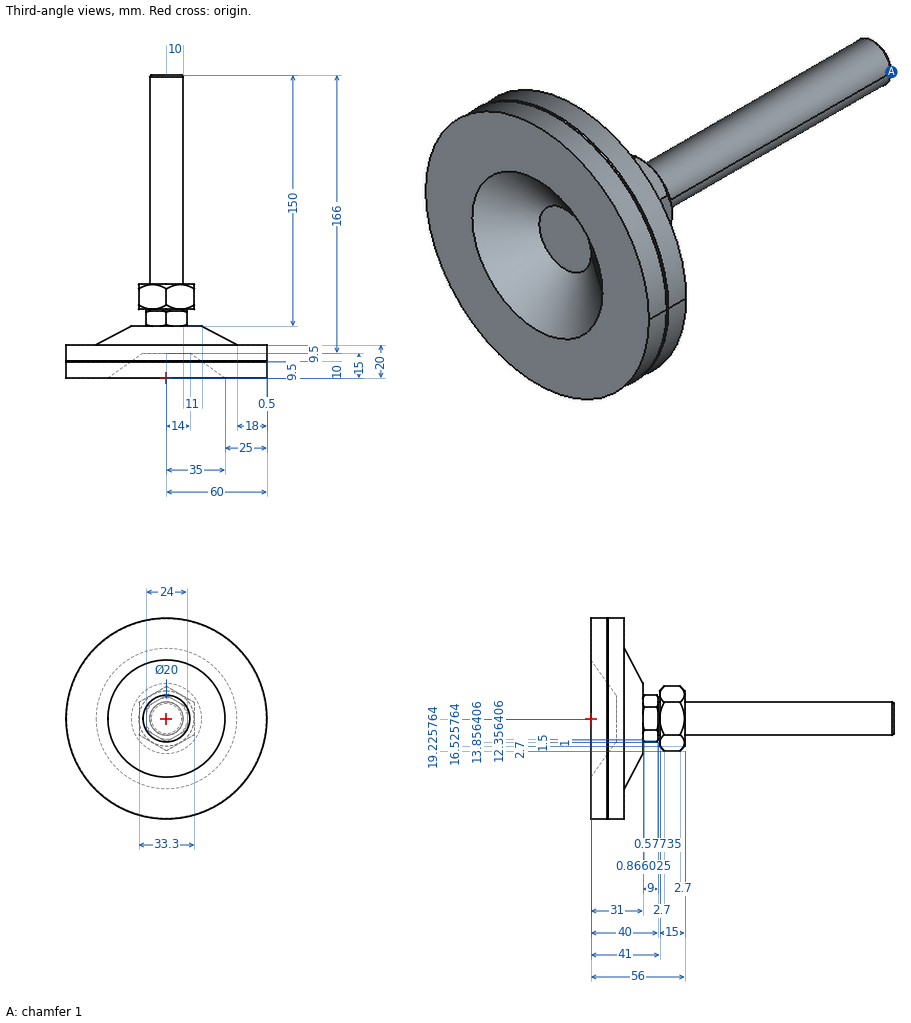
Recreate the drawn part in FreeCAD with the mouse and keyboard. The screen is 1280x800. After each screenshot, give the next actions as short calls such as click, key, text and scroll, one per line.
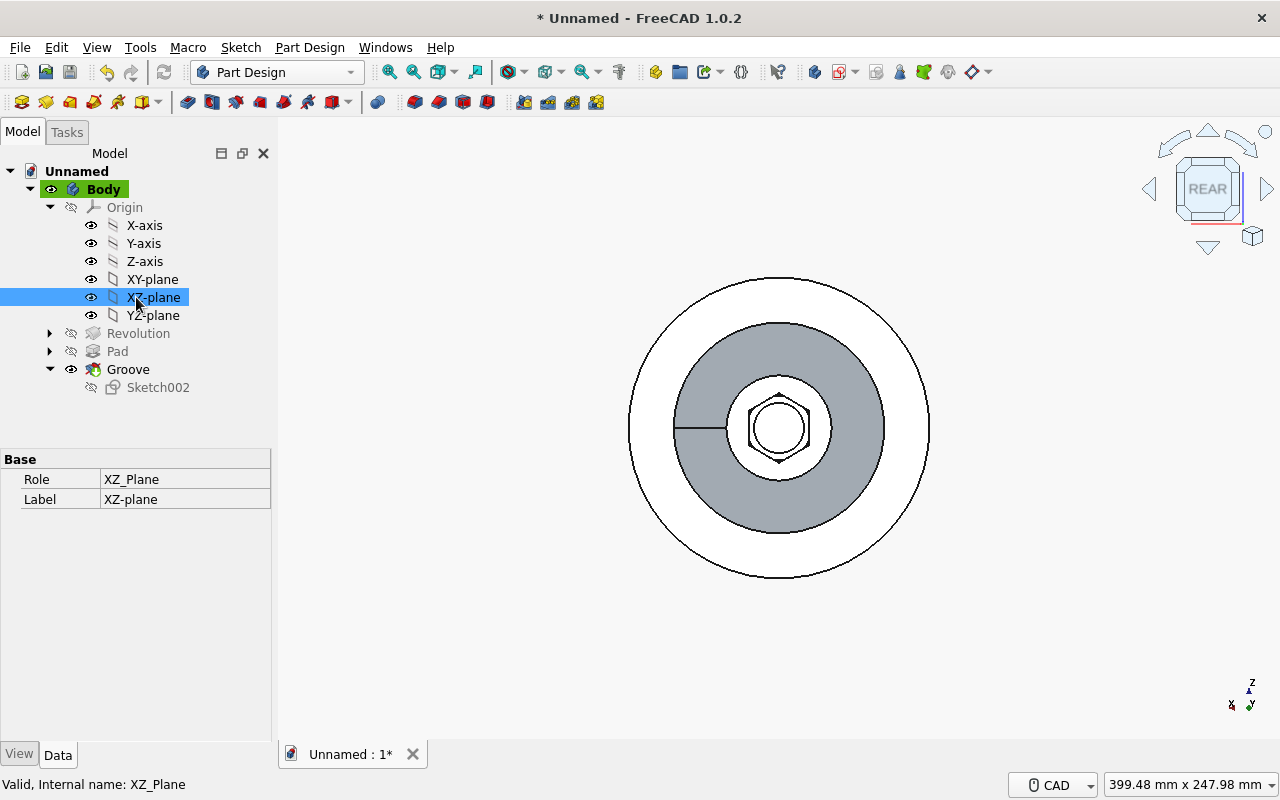
click(972, 72)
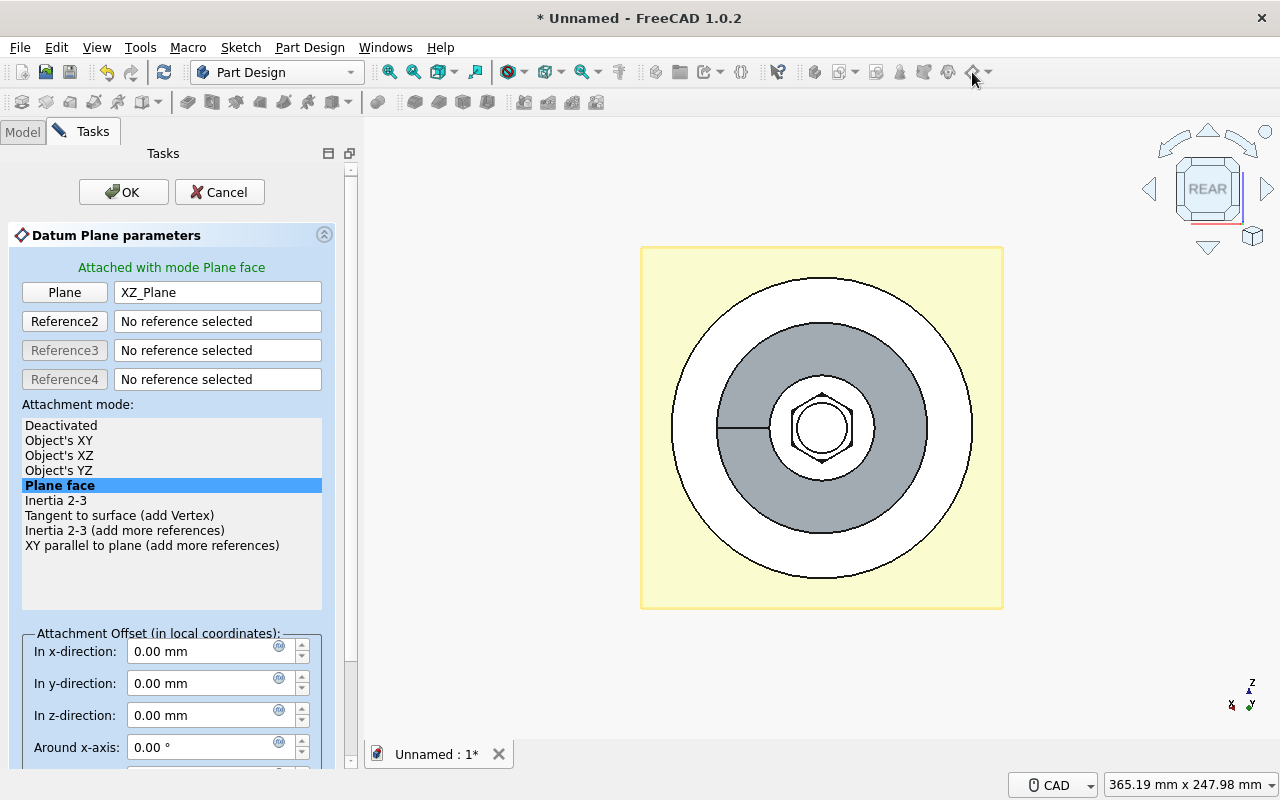
triple_click(210, 715)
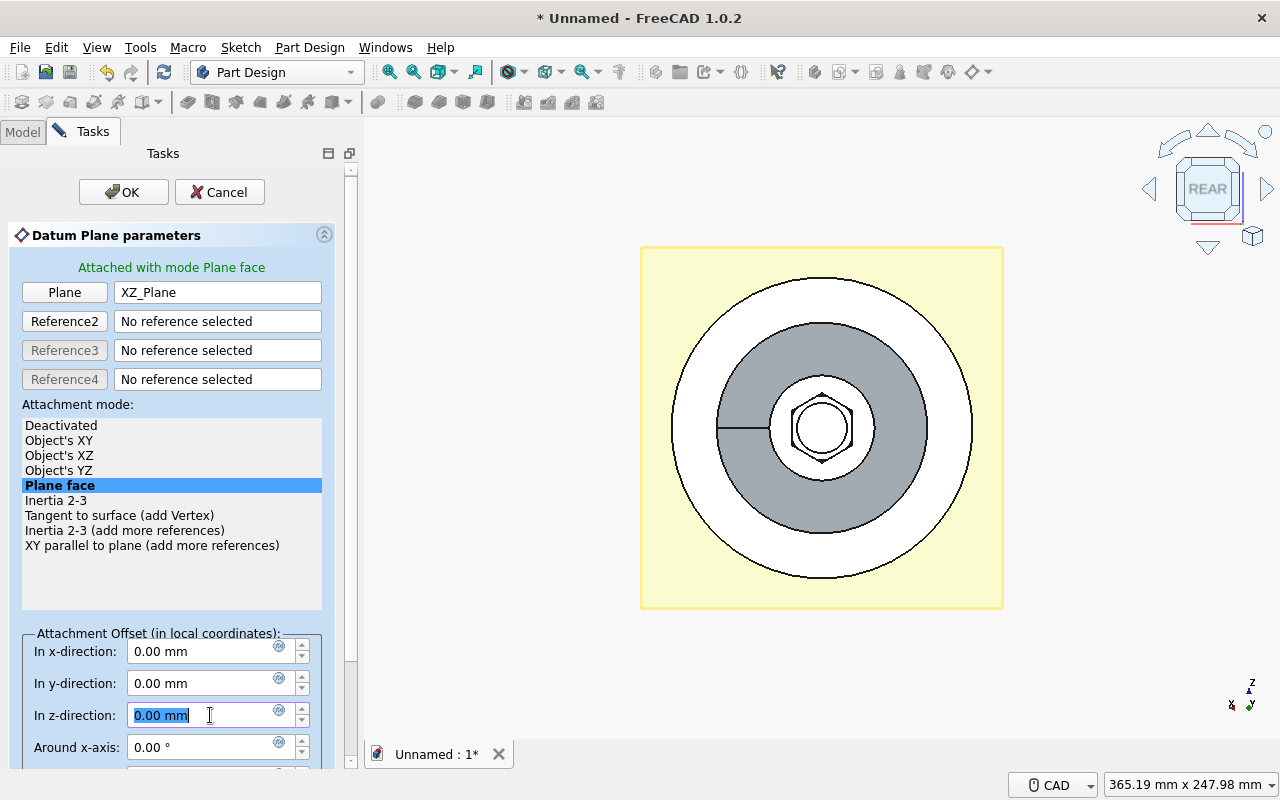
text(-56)
key(Tab)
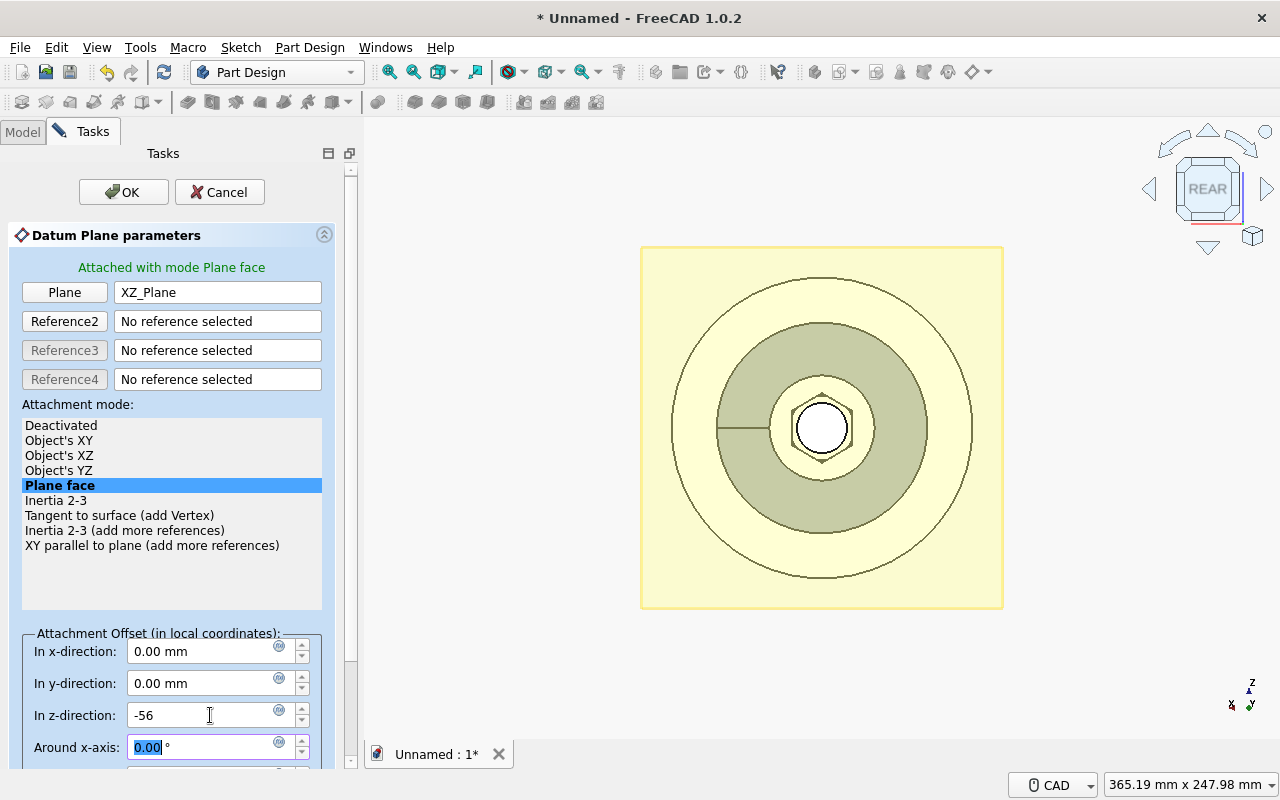
click(124, 192)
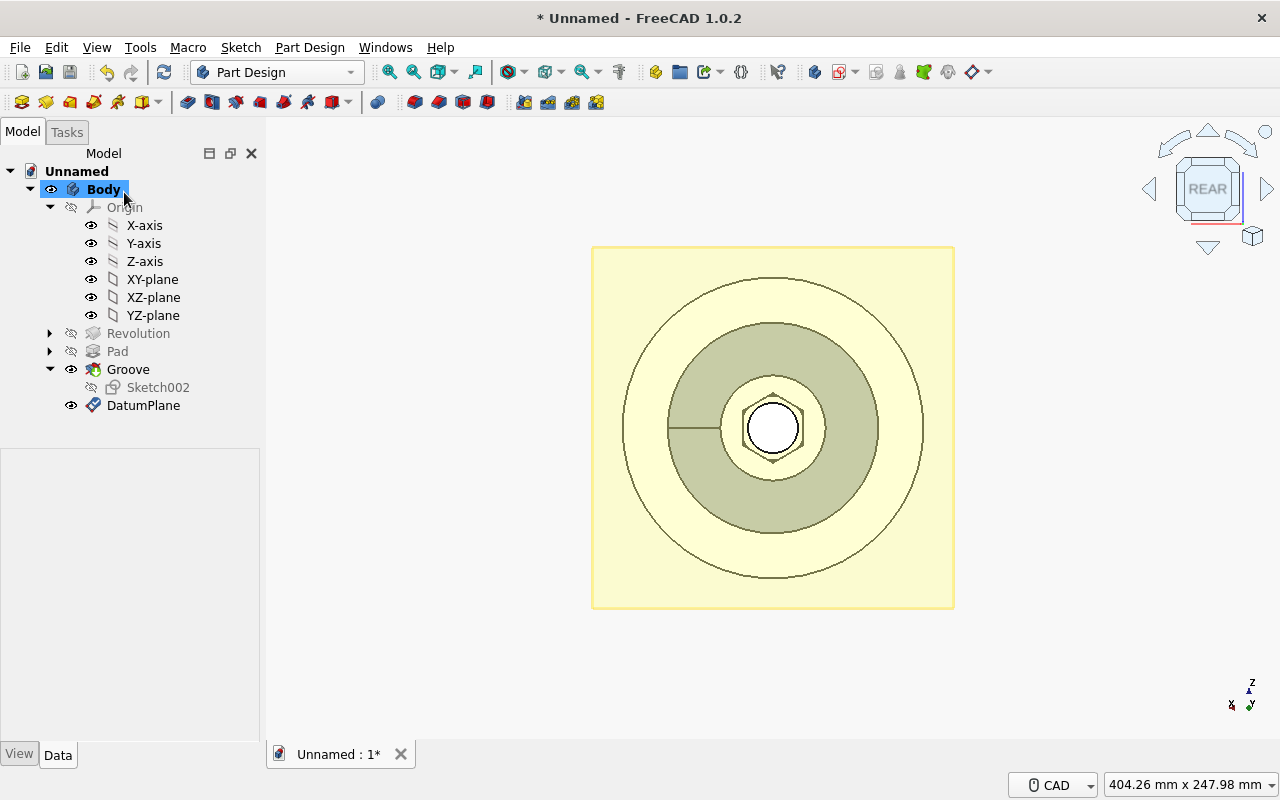
click(116, 405)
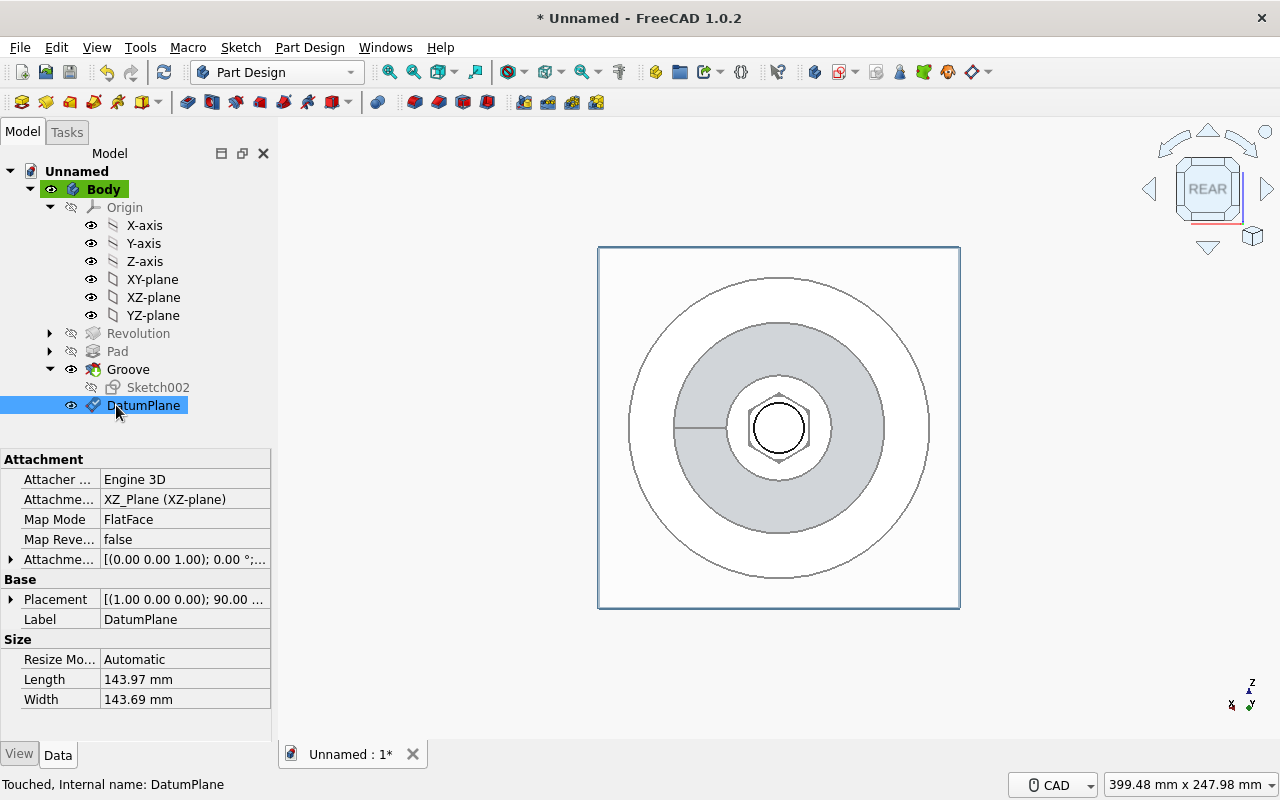
click(840, 72)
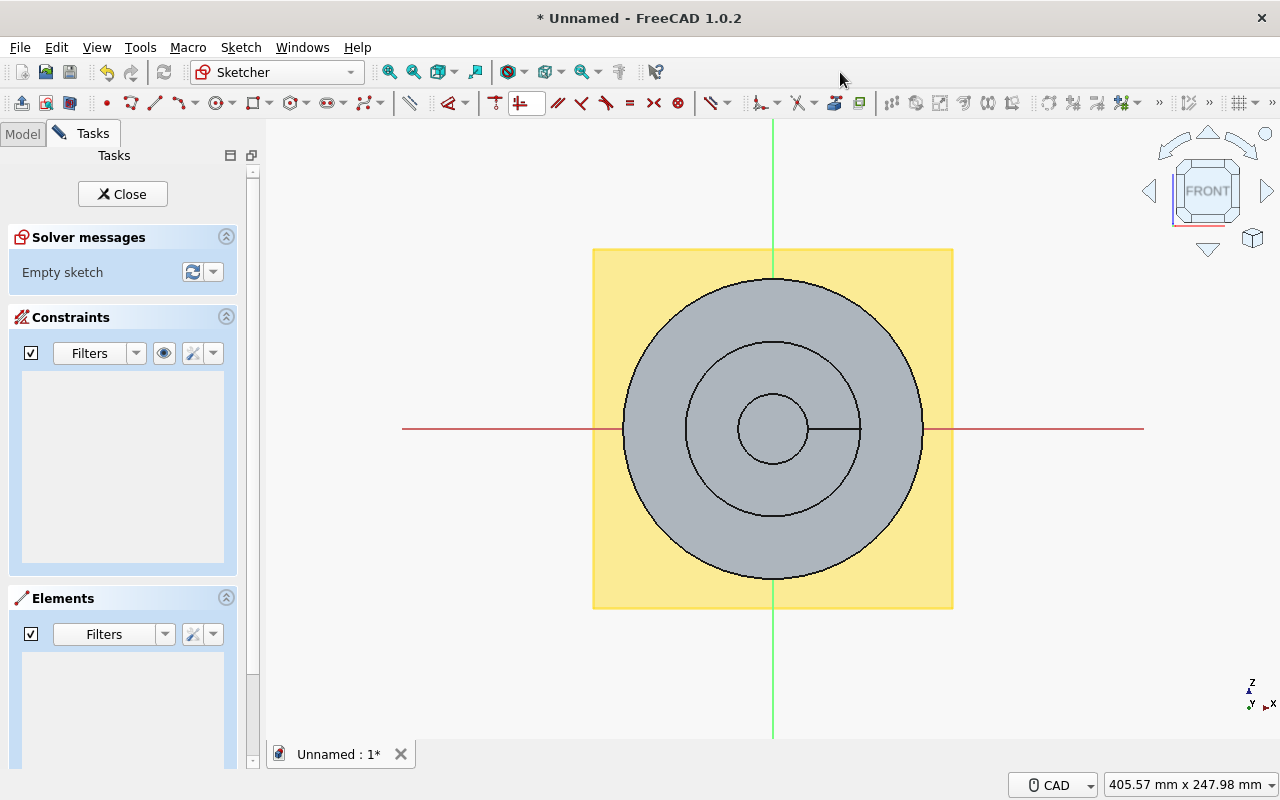
click(70, 104)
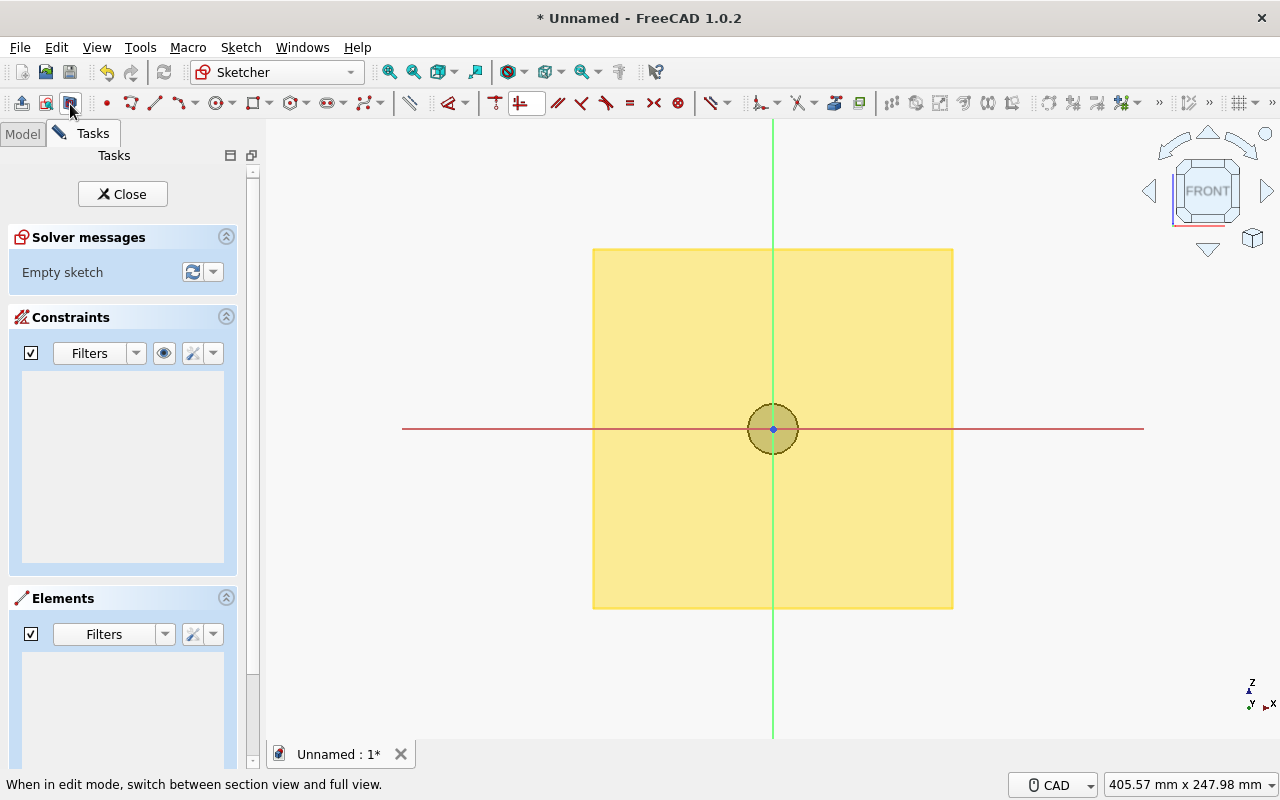
scroll(795, 429, up, 7)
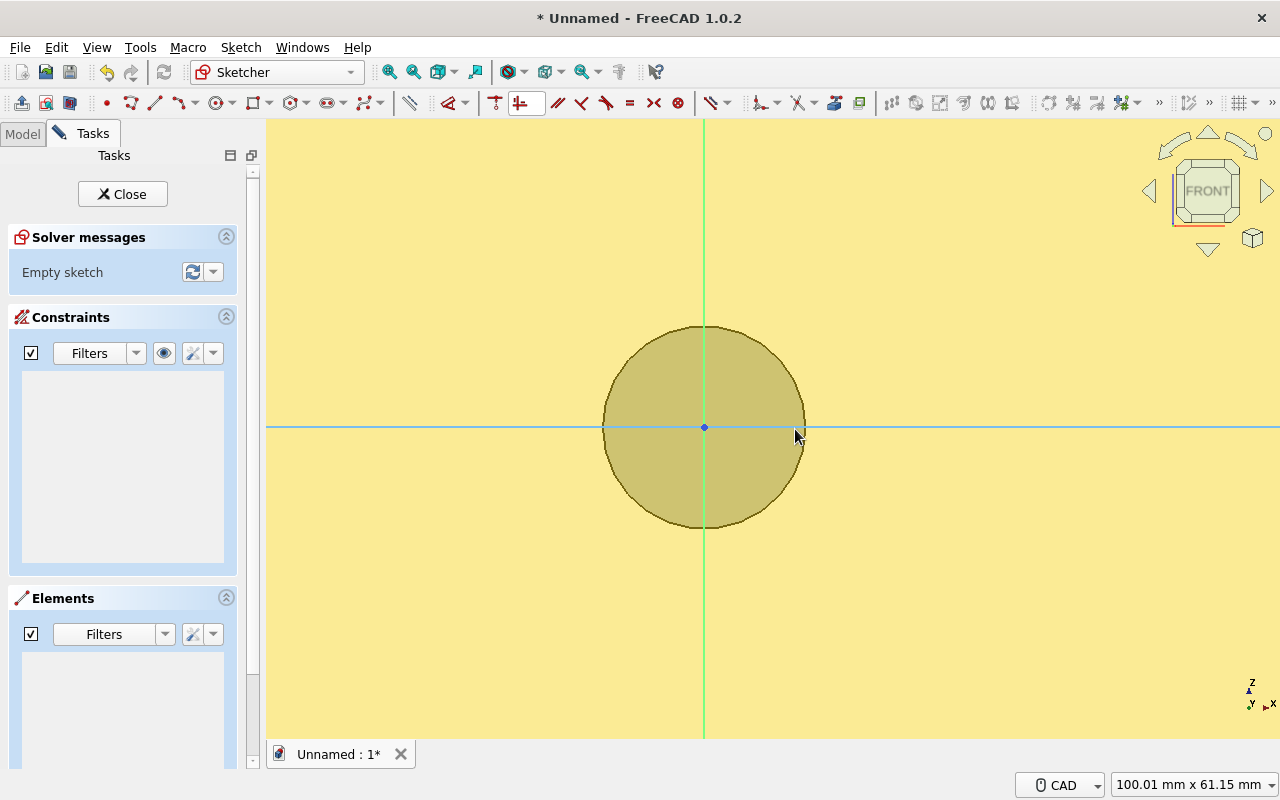
click(290, 104)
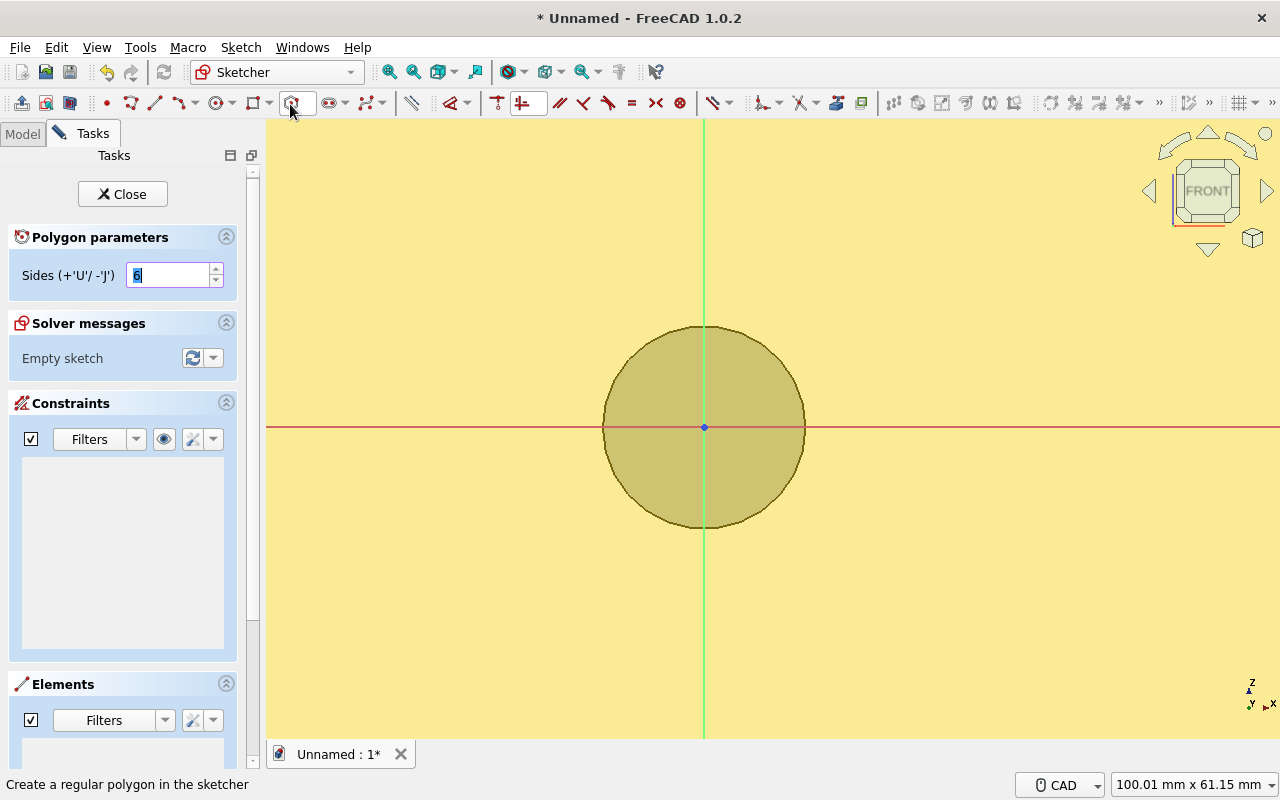
click(704, 427)